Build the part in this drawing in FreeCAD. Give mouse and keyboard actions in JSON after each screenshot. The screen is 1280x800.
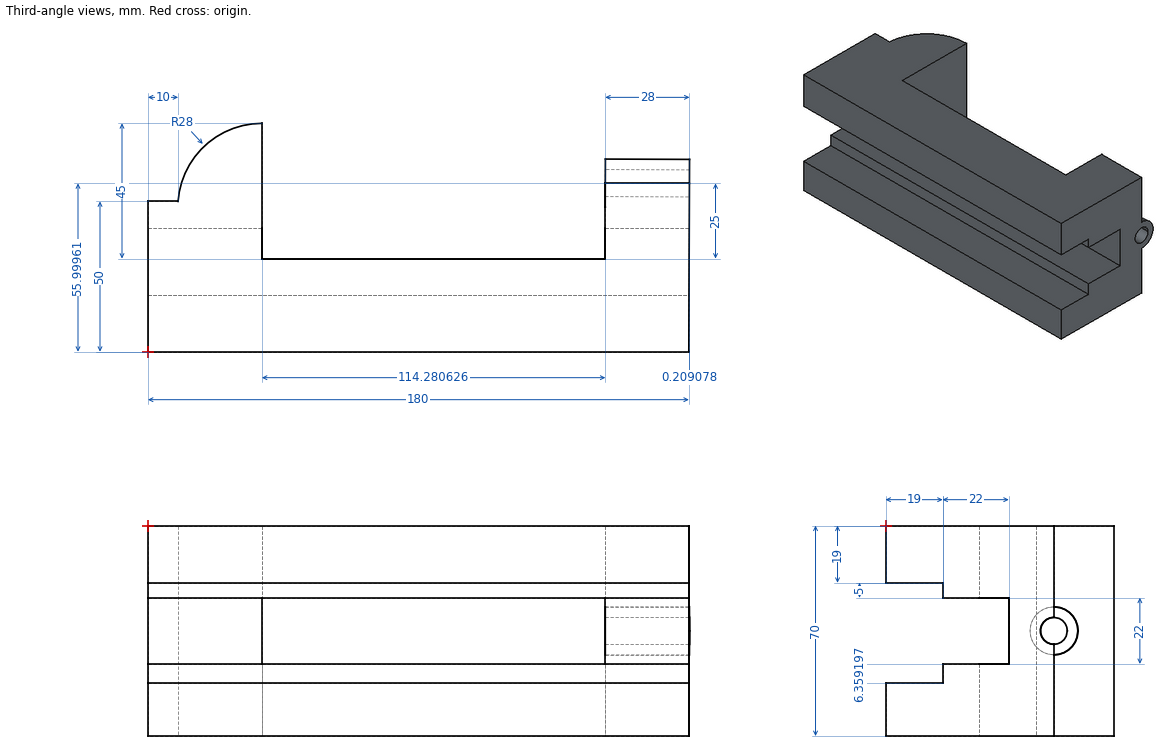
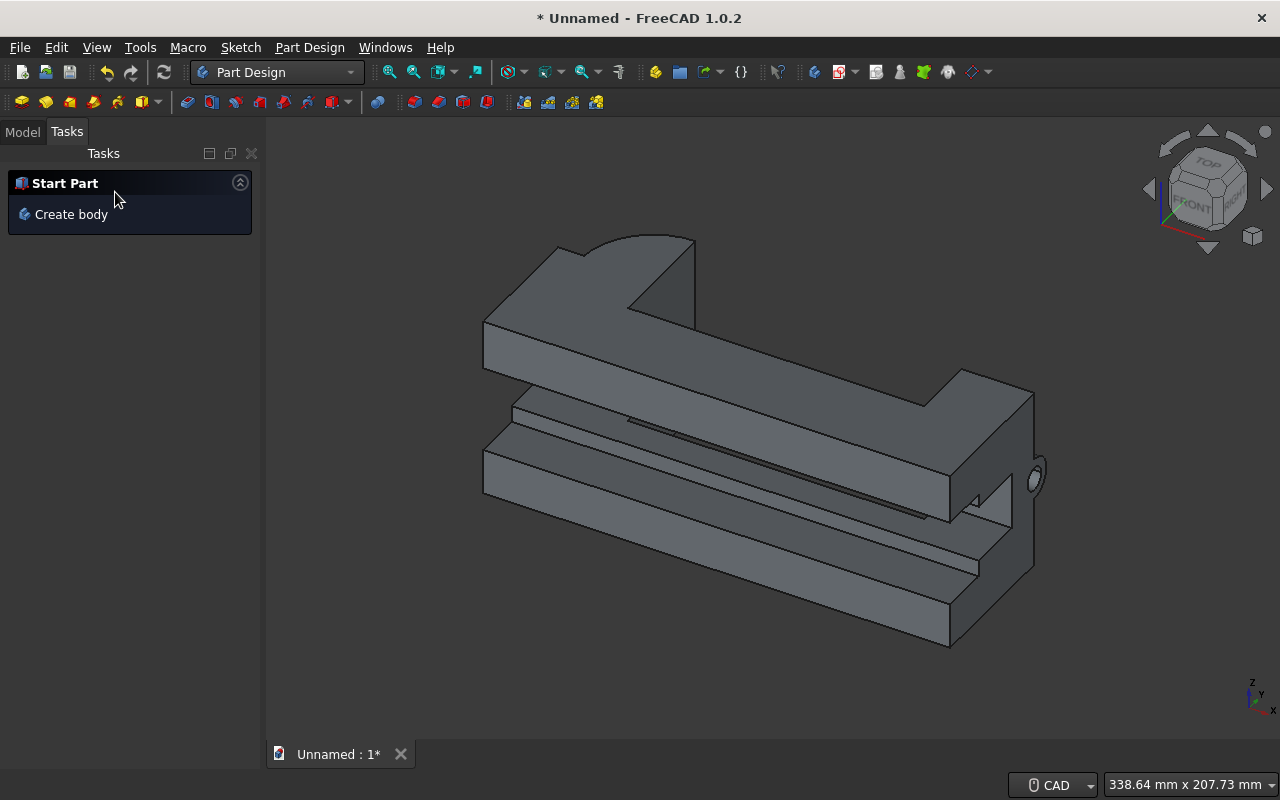
{"action": "key", "text": "0"}